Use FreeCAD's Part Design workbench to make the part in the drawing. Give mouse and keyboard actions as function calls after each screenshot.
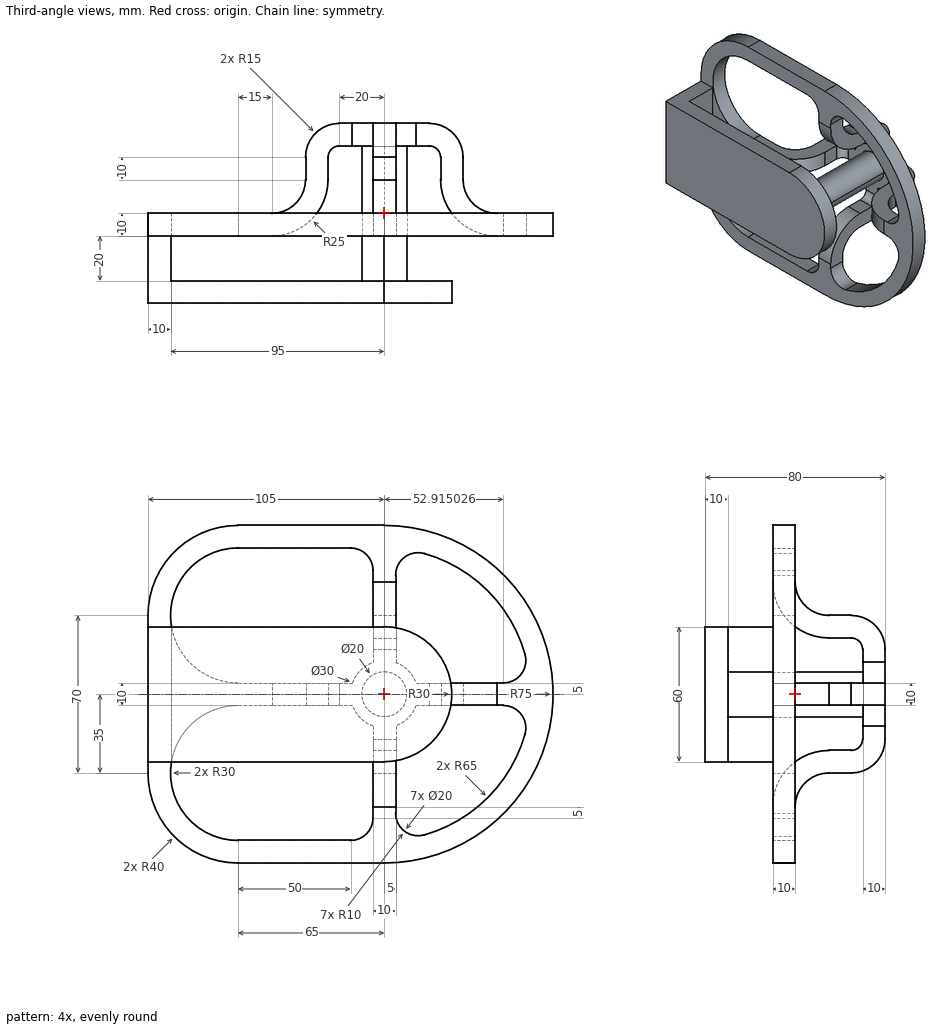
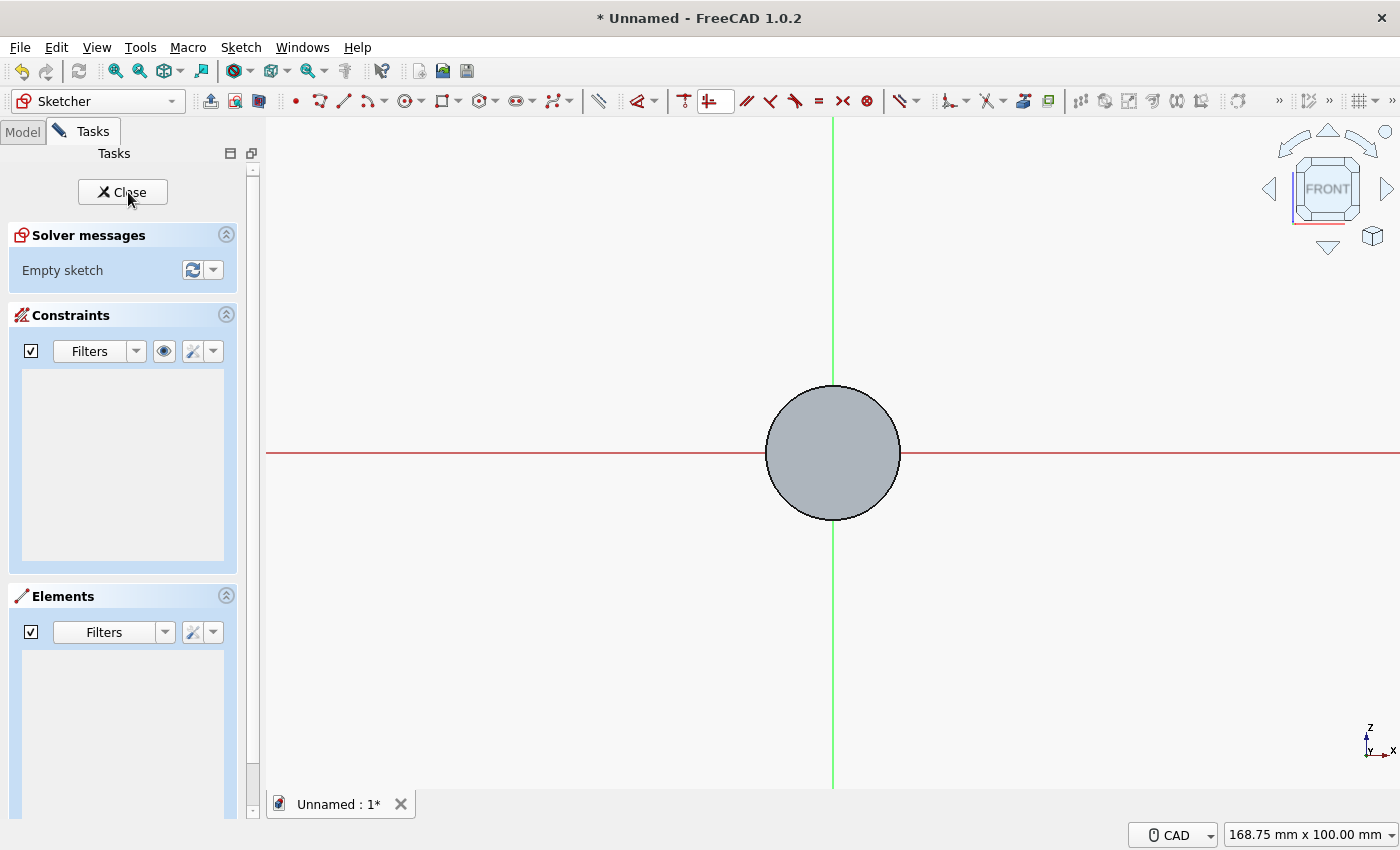
click(260, 102)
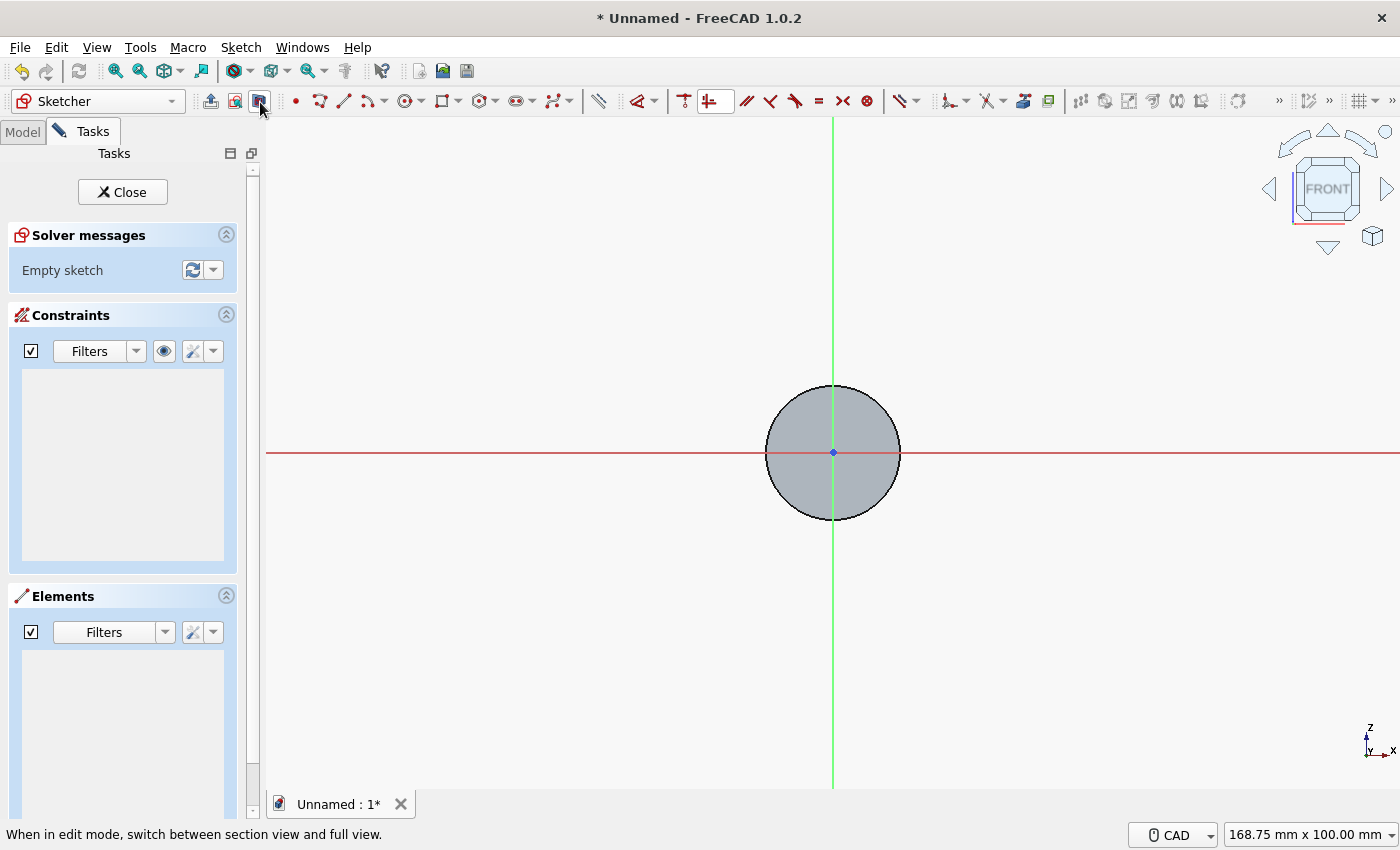
scroll(791, 453, down, 4)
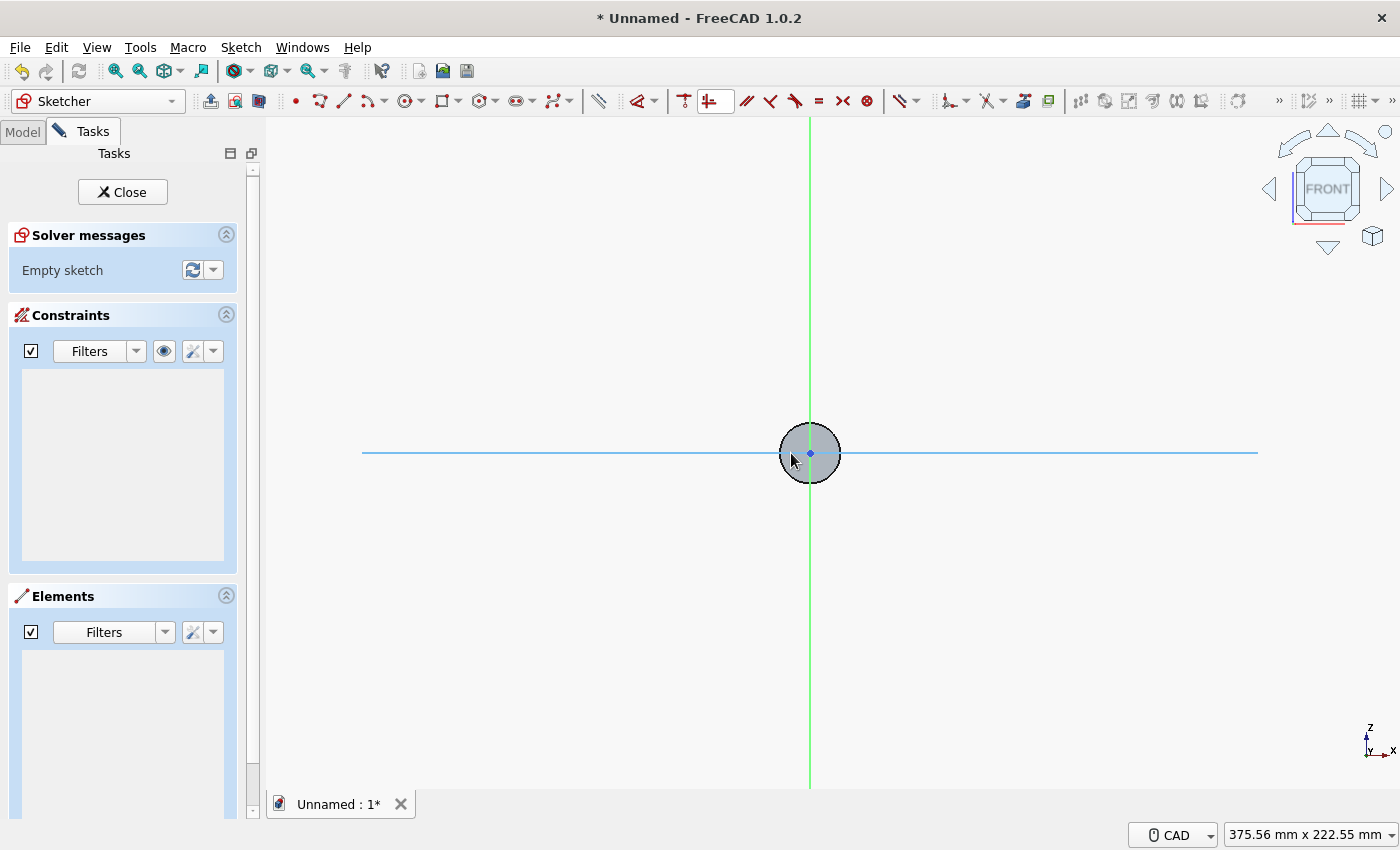
click(344, 102)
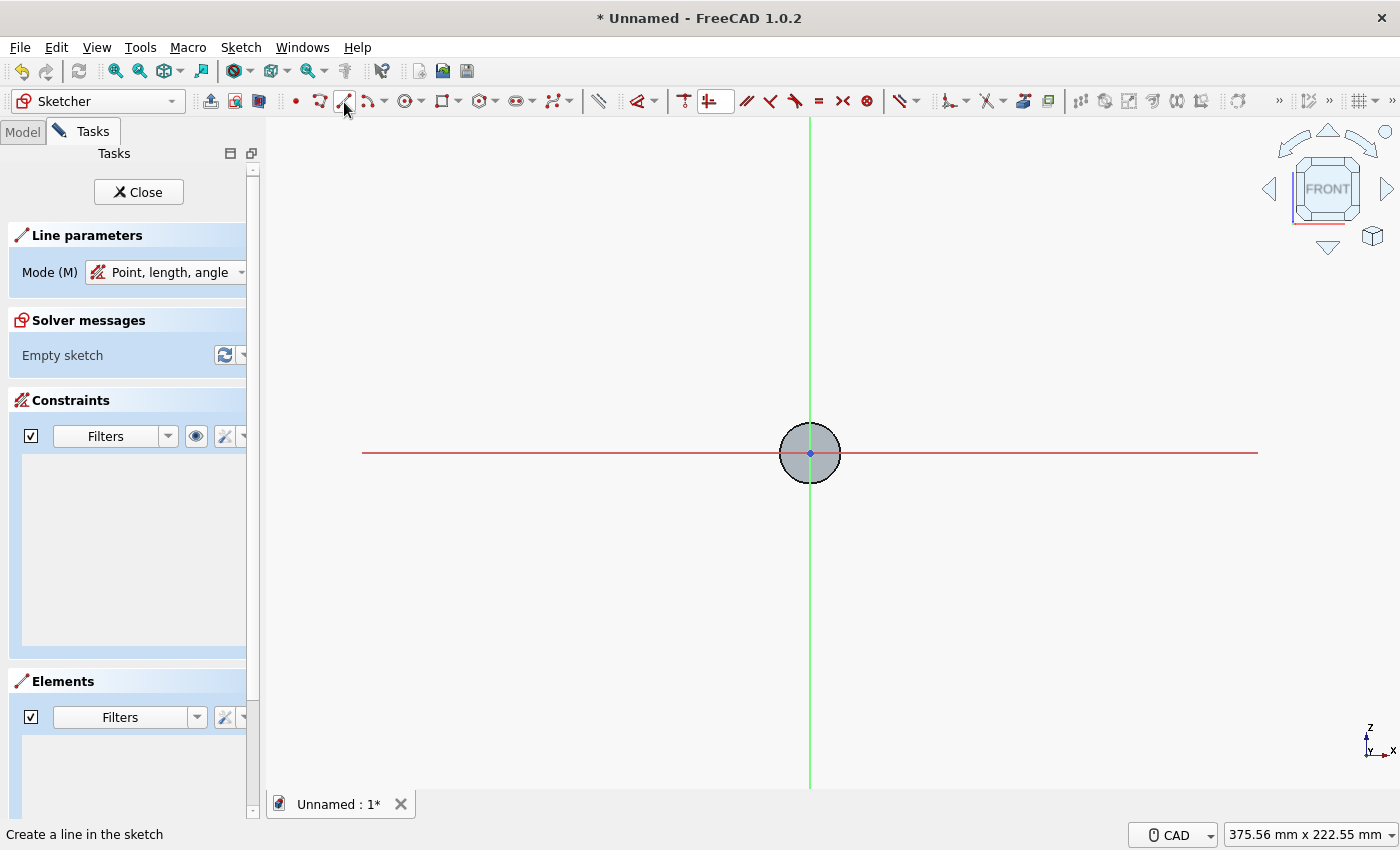
click(810, 680)
click(614, 680)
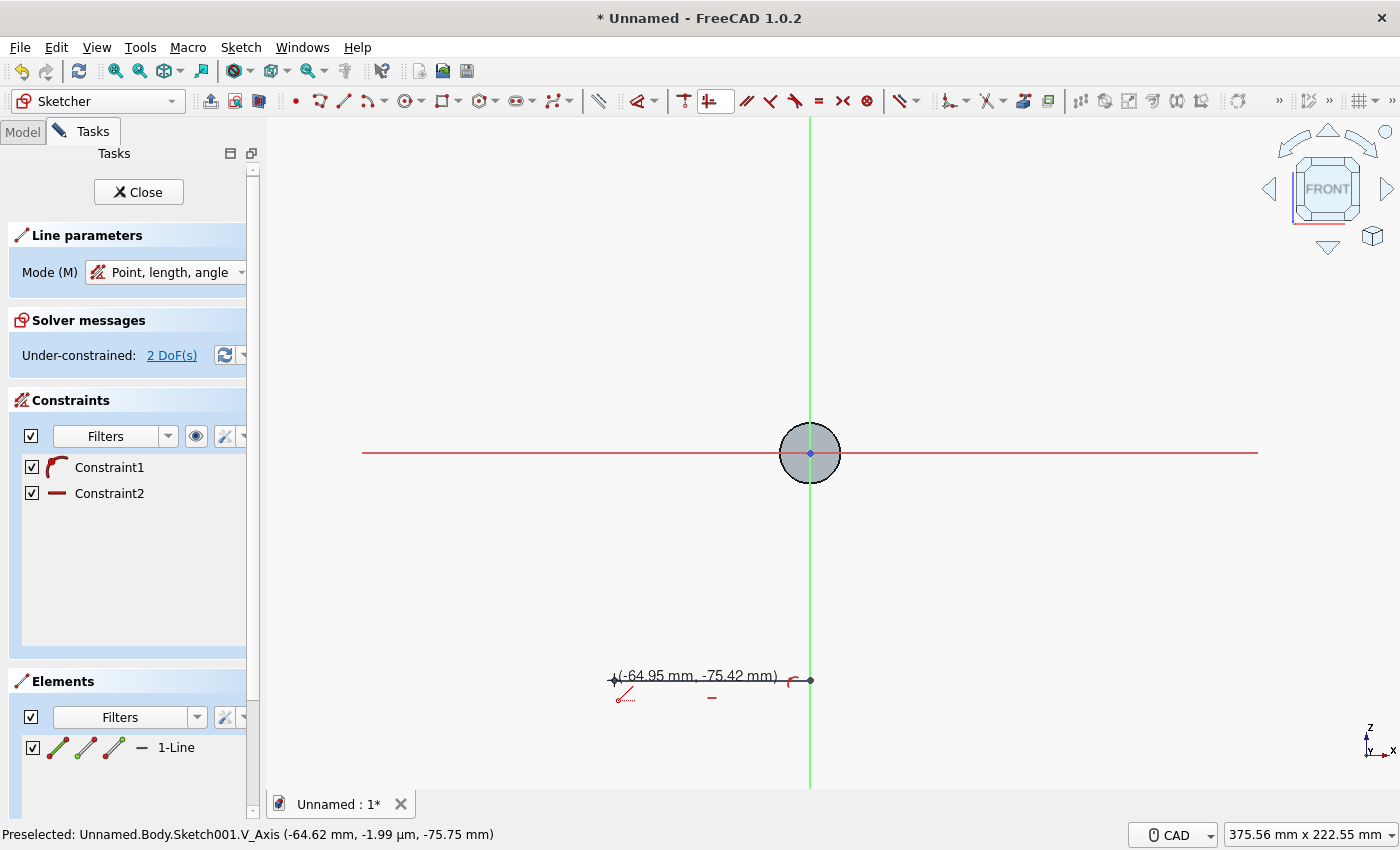
click(493, 559)
click(493, 348)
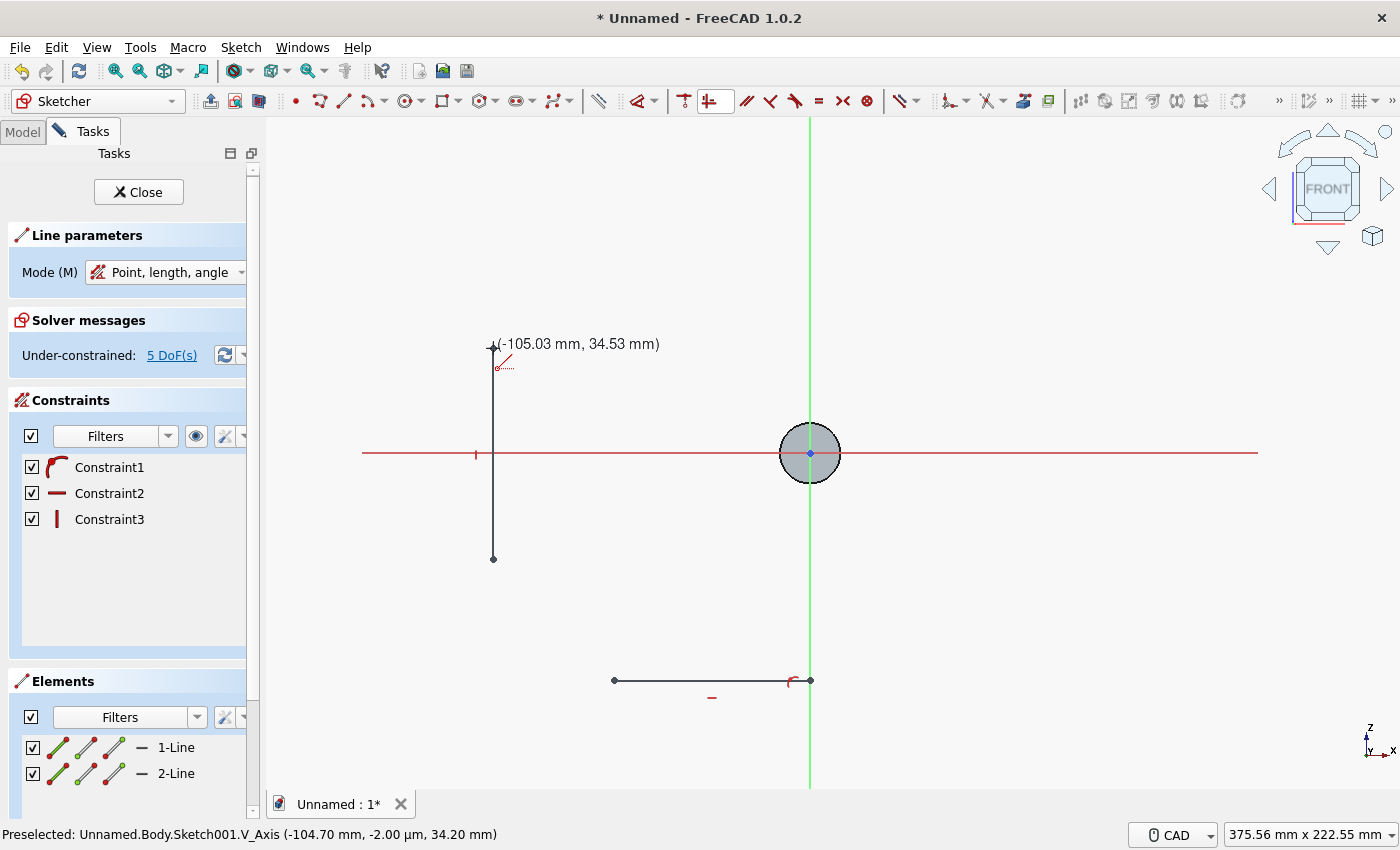
click(614, 227)
click(810, 227)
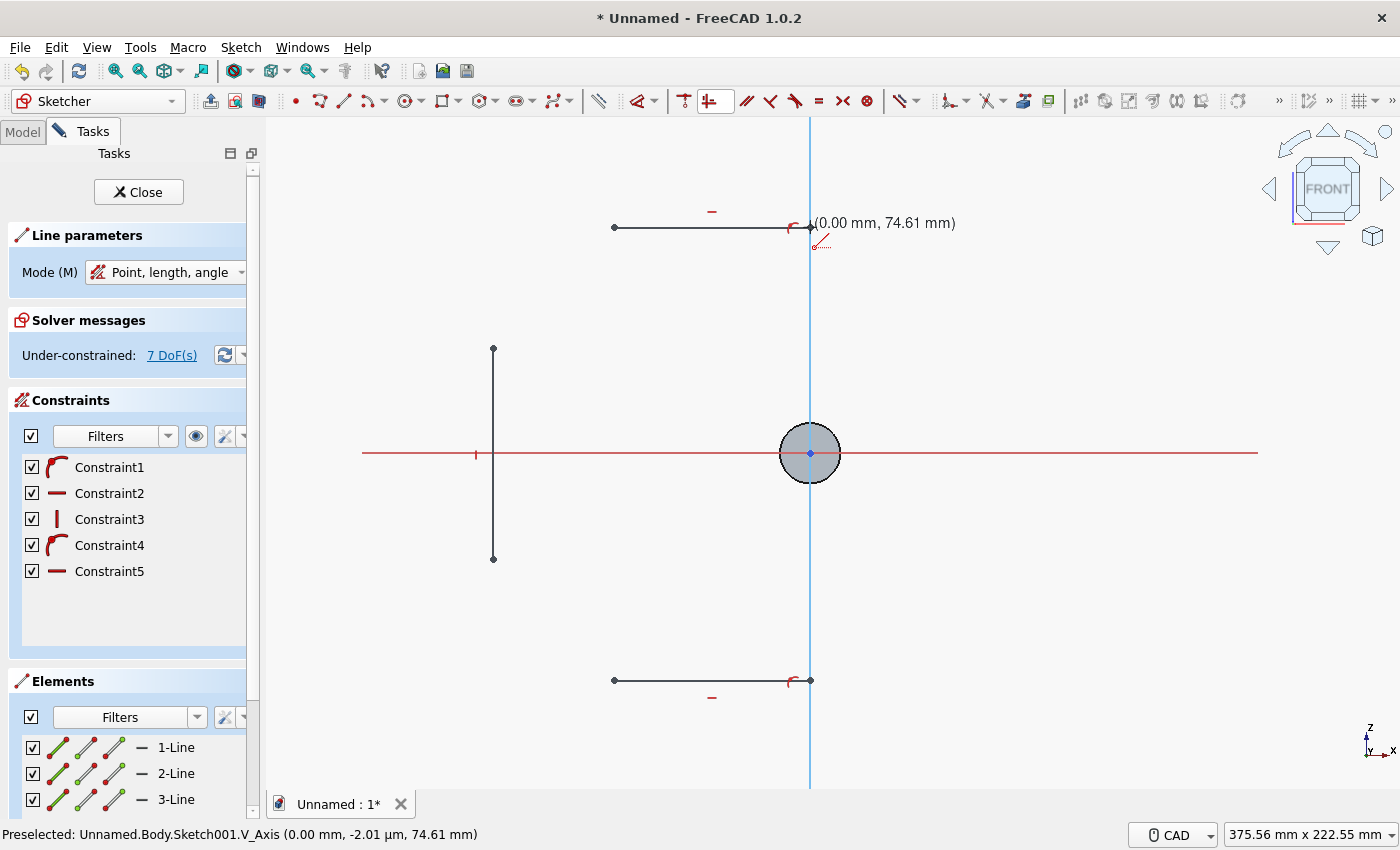
click(386, 102)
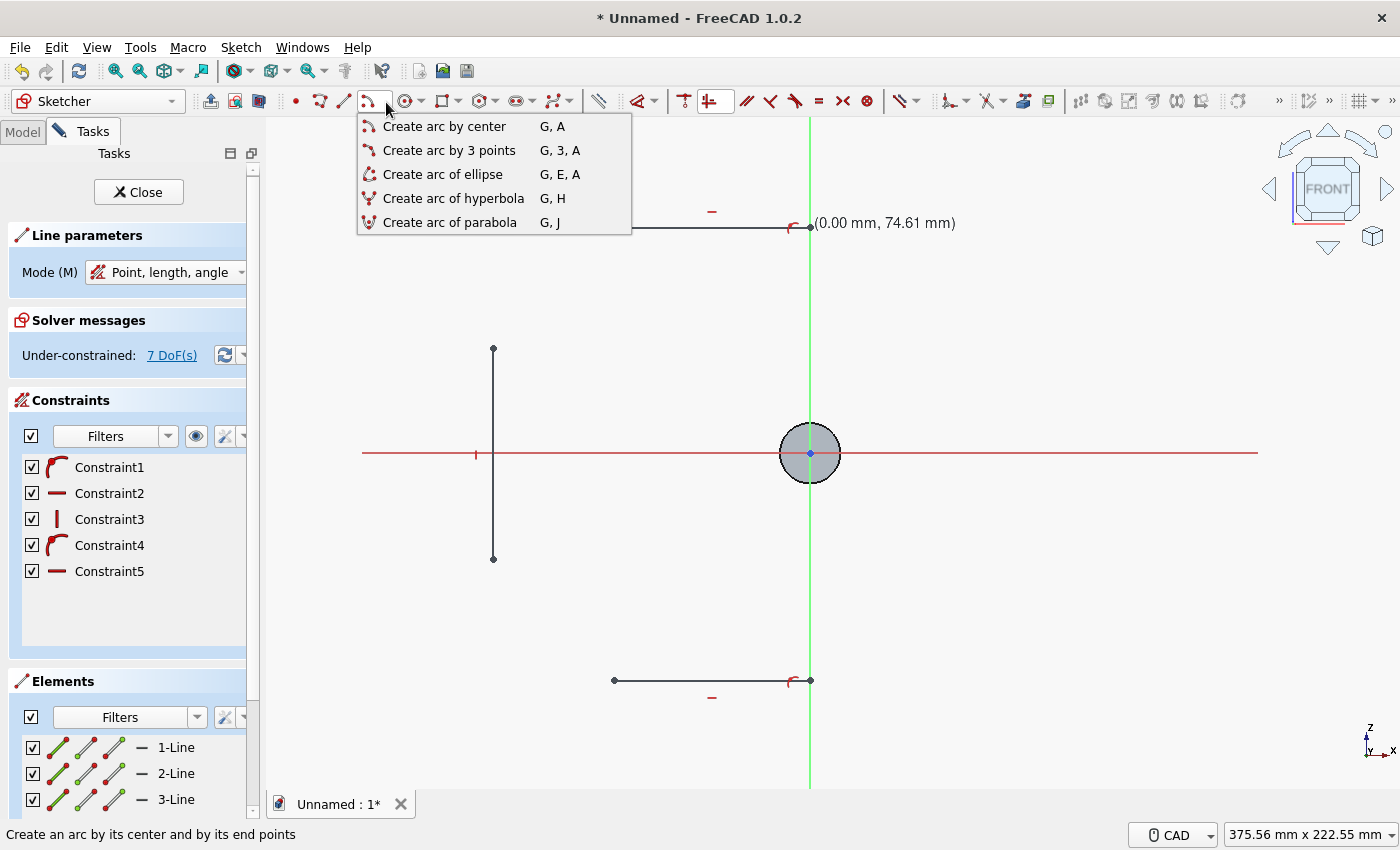
click(494, 150)